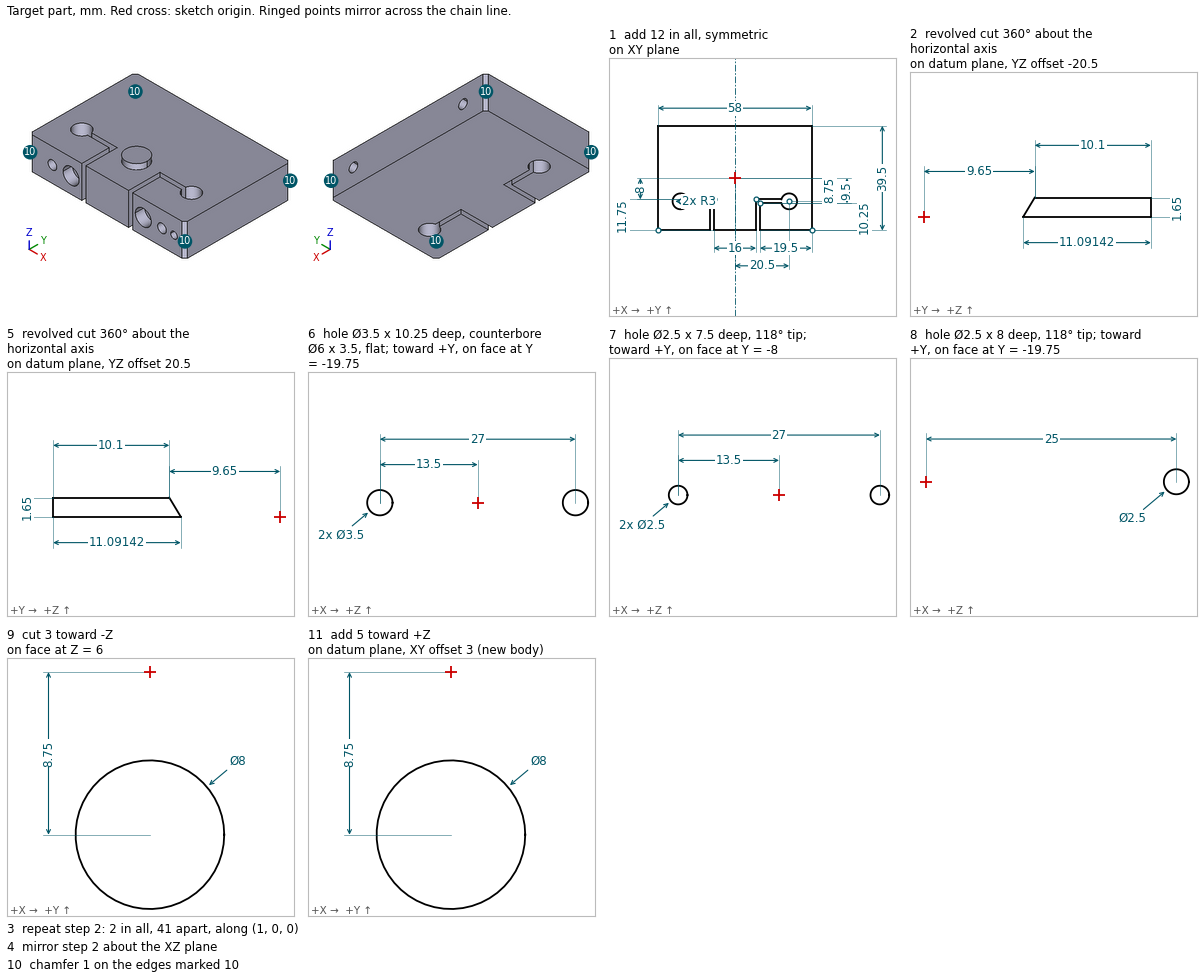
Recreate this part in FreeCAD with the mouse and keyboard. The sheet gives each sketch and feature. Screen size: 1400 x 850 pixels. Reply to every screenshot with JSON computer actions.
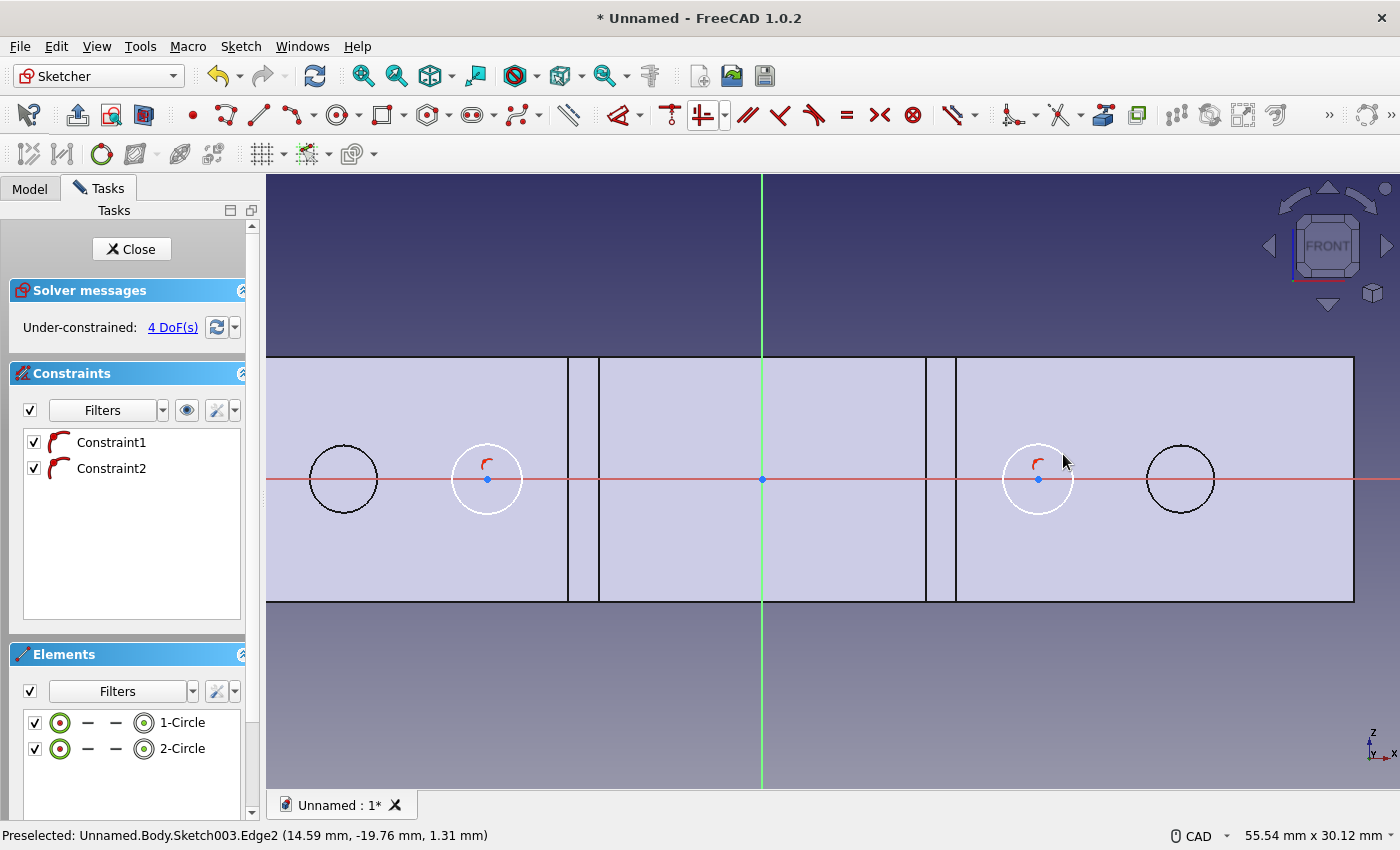
{"action": "left_click", "coordinate": [512, 455]}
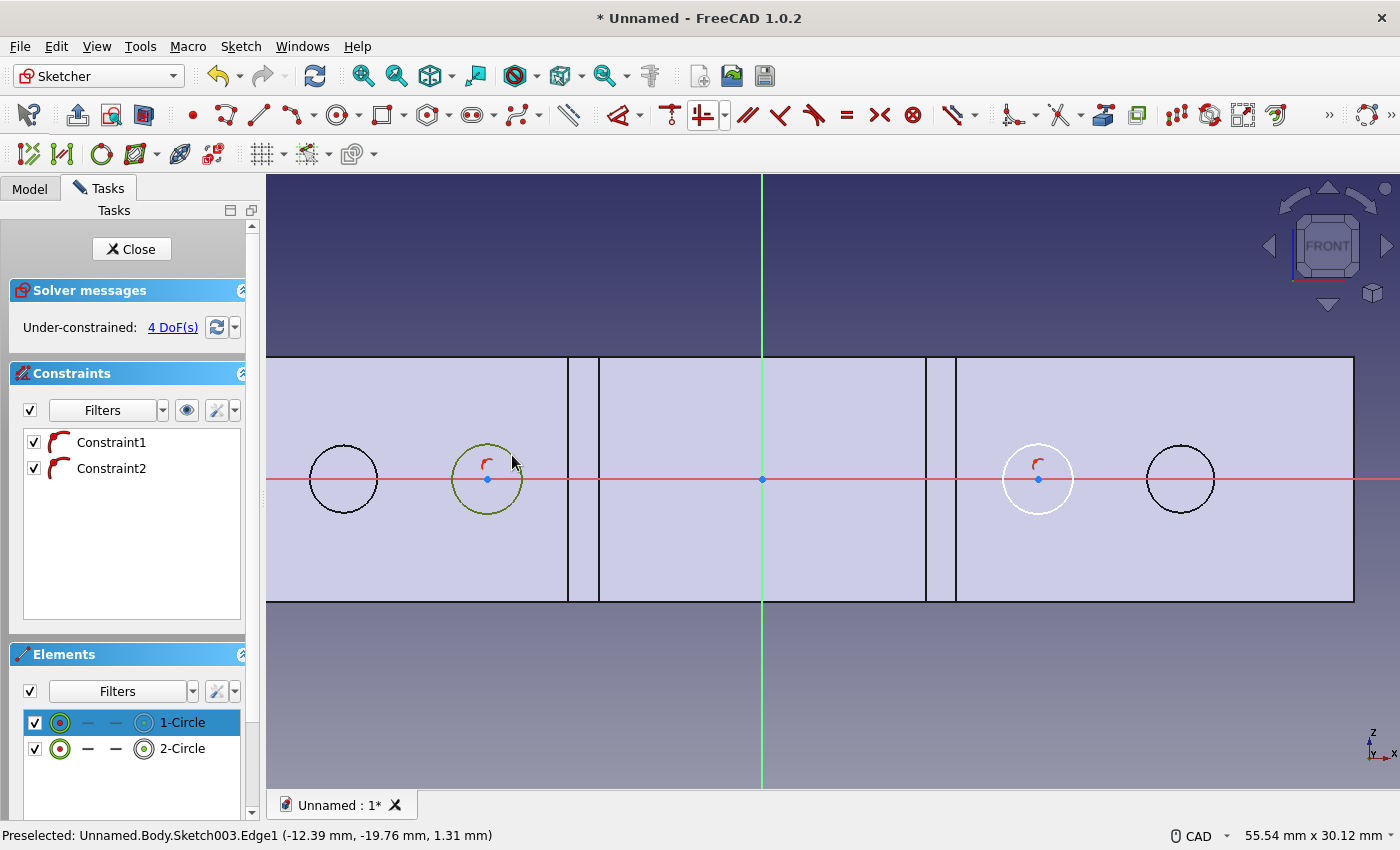
{"action": "left_click", "coordinate": [1063, 455]}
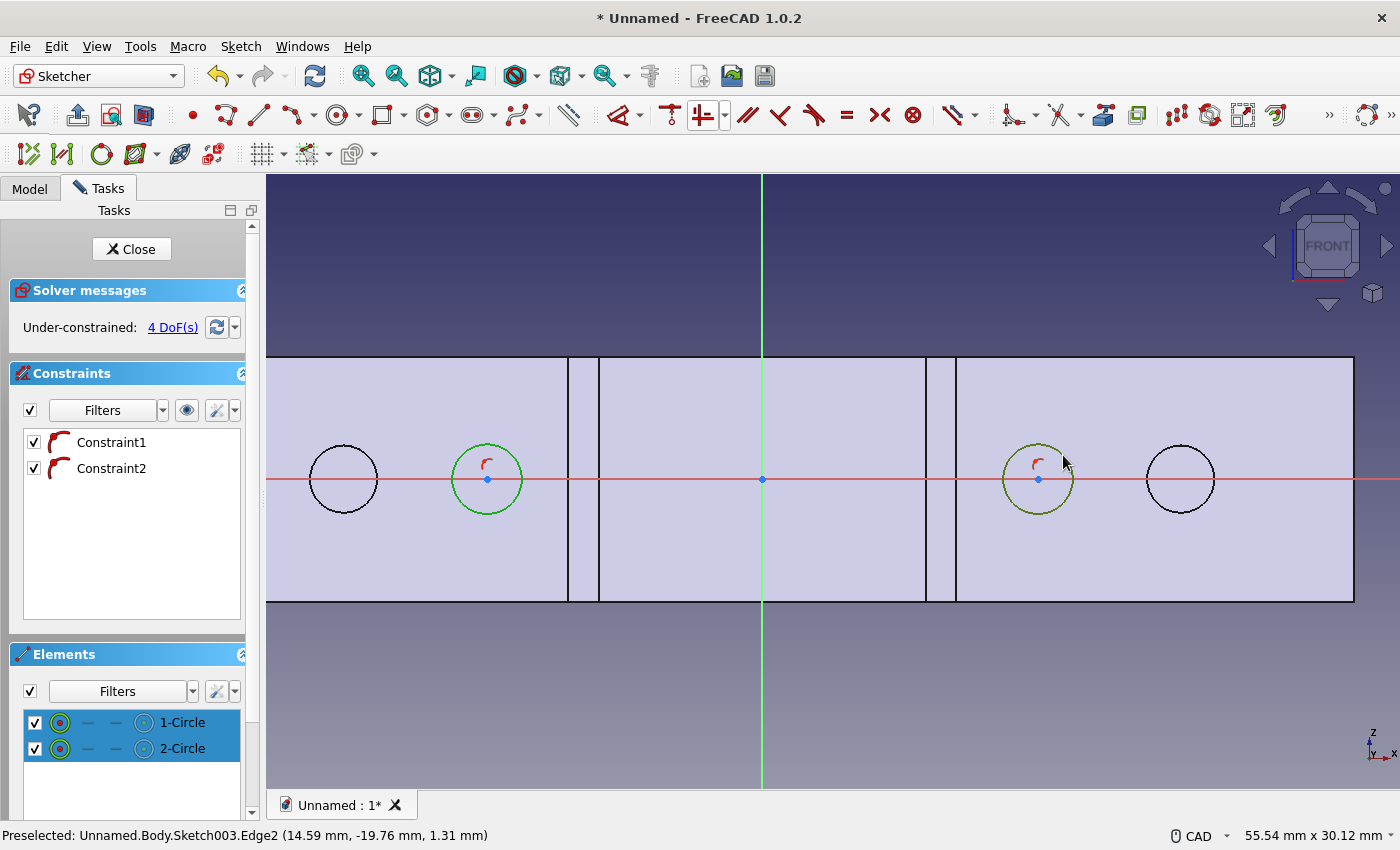
{"action": "left_click", "coordinate": [847, 116]}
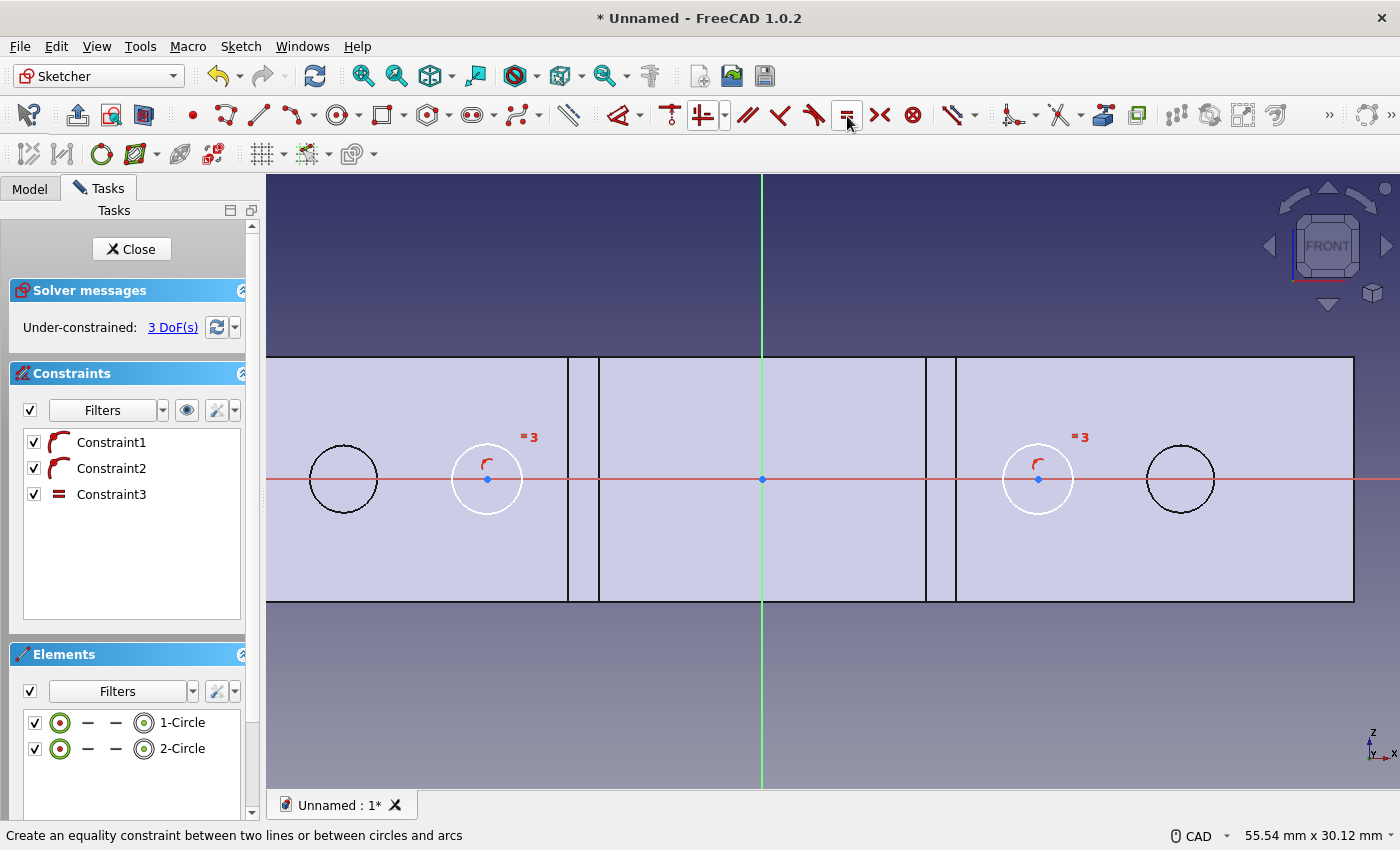
{"action": "left_click", "coordinate": [618, 116]}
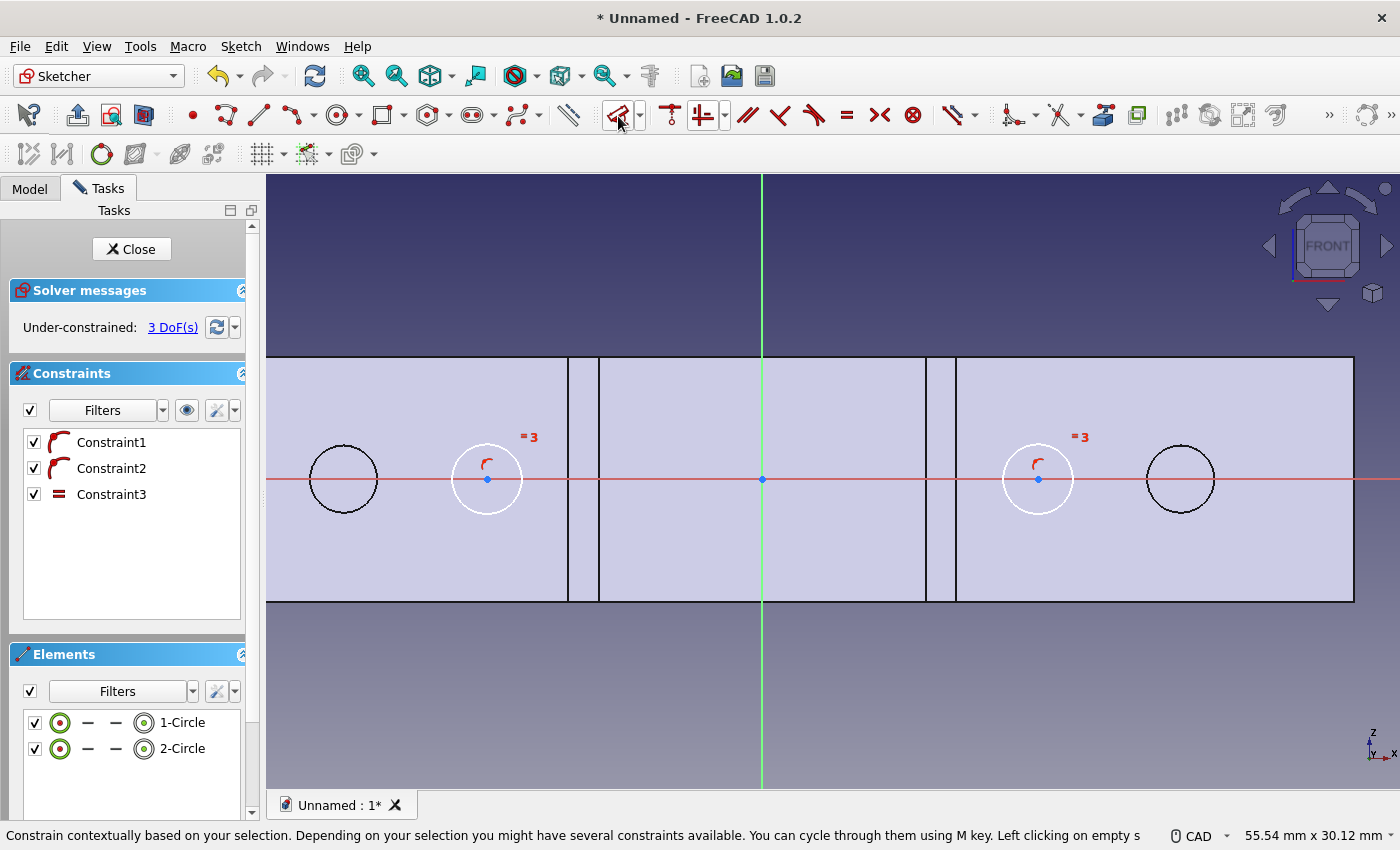
{"action": "left_click", "coordinate": [512, 455]}
{"action": "left_click", "coordinate": [535, 433]}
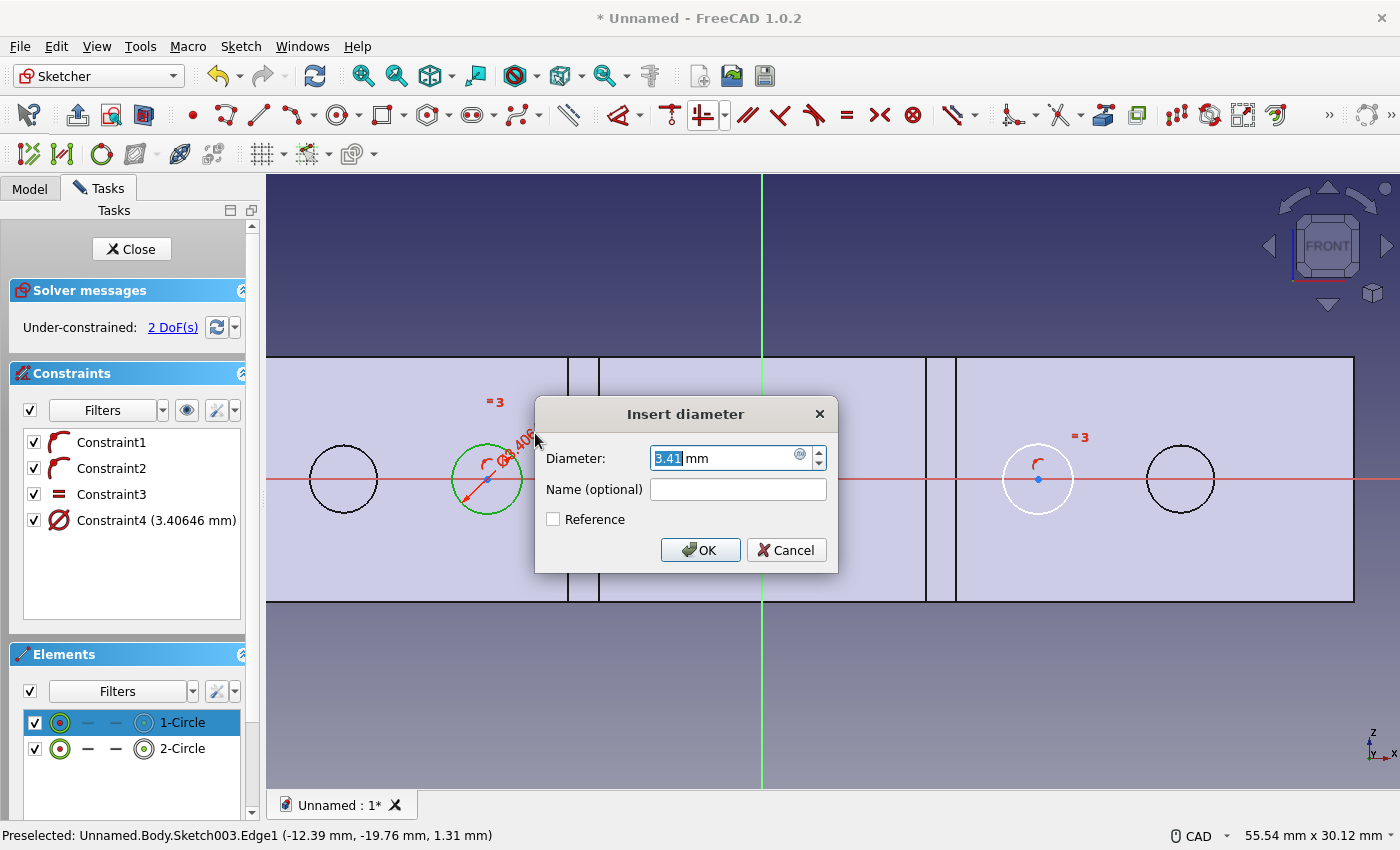
{"action": "type", "text": "3.5"}
{"action": "key", "text": "Return"}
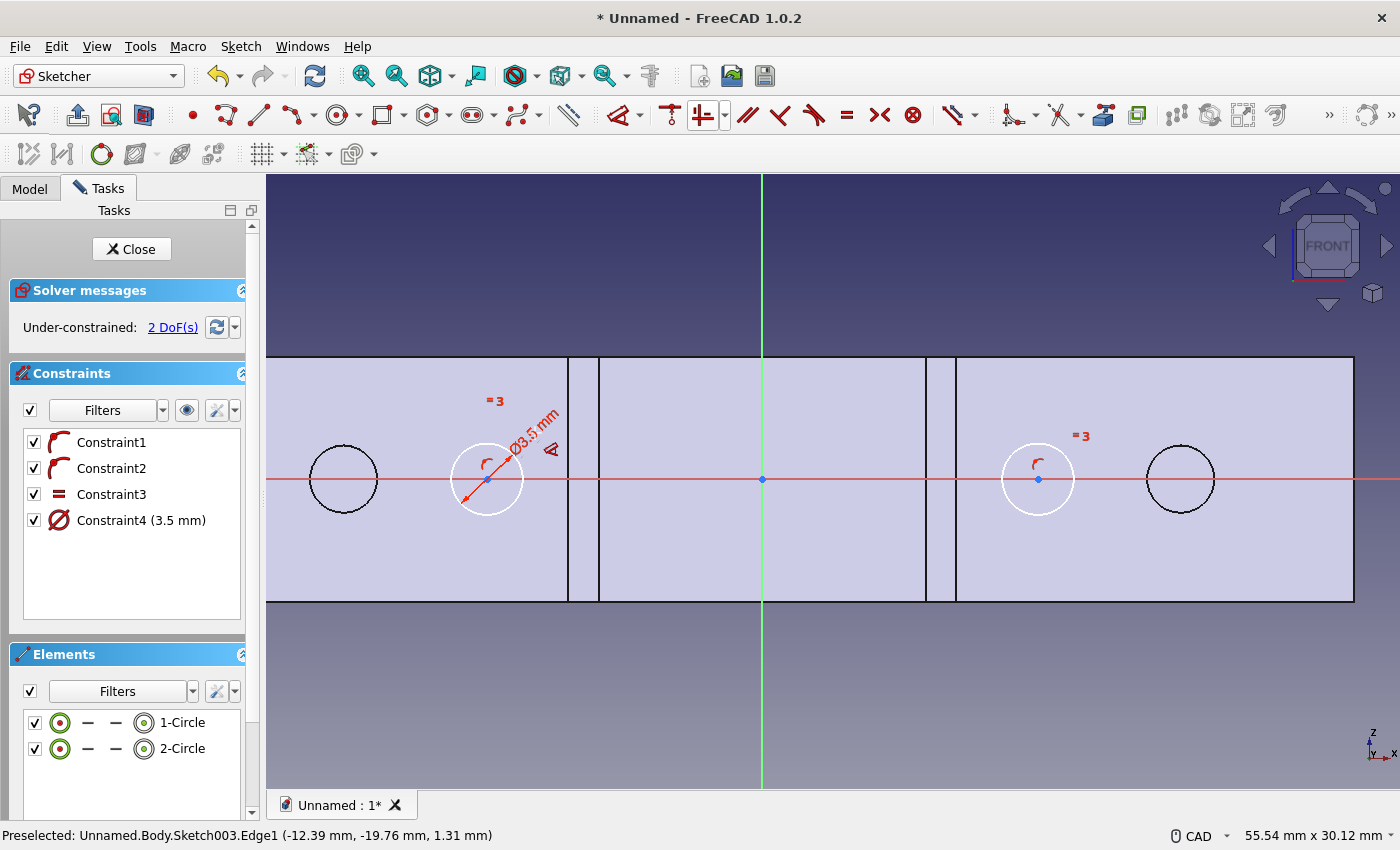
{"action": "left_click", "coordinate": [487, 479]}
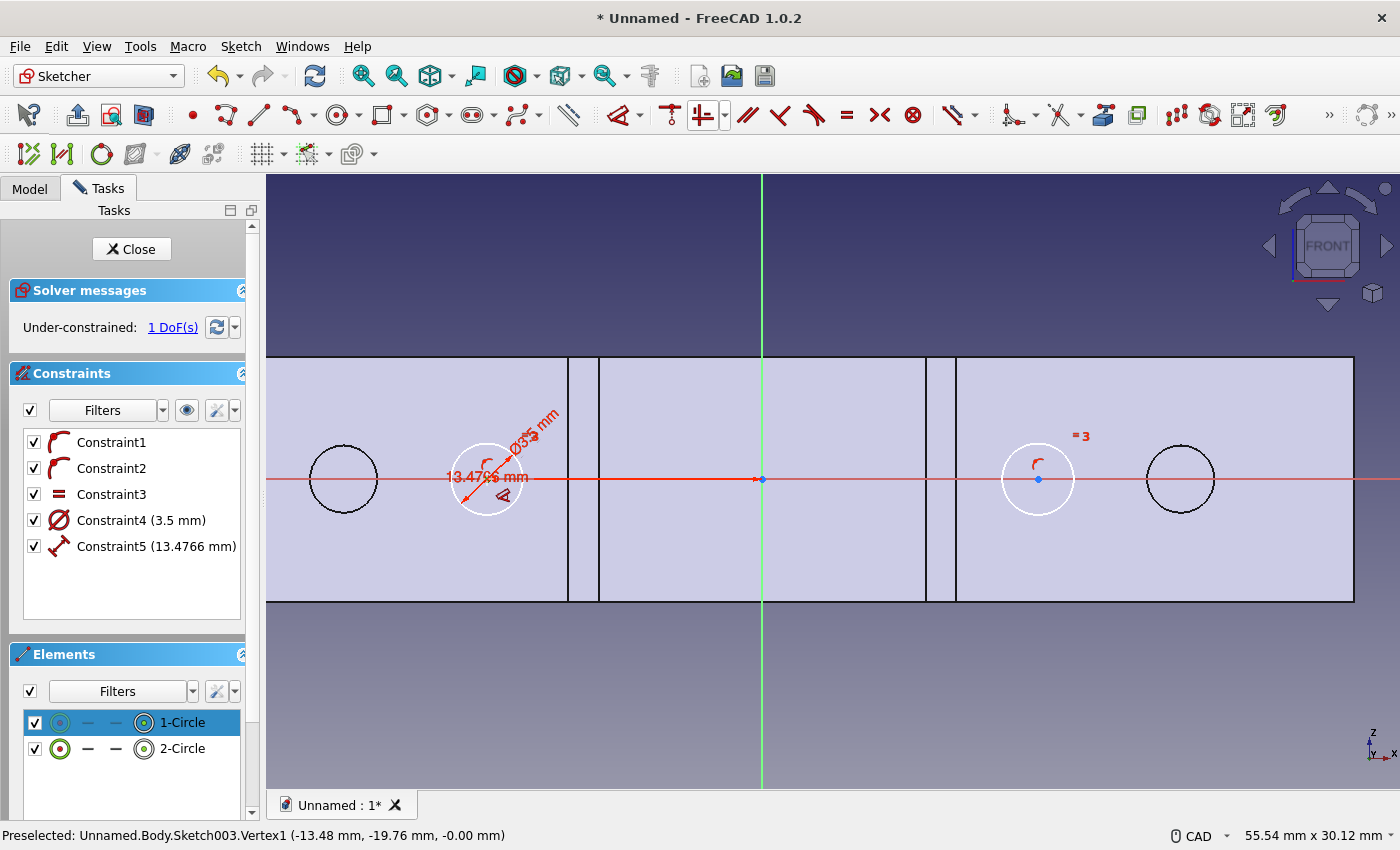
{"action": "left_click", "coordinate": [1038, 479]}
{"action": "left_click", "coordinate": [636, 513]}